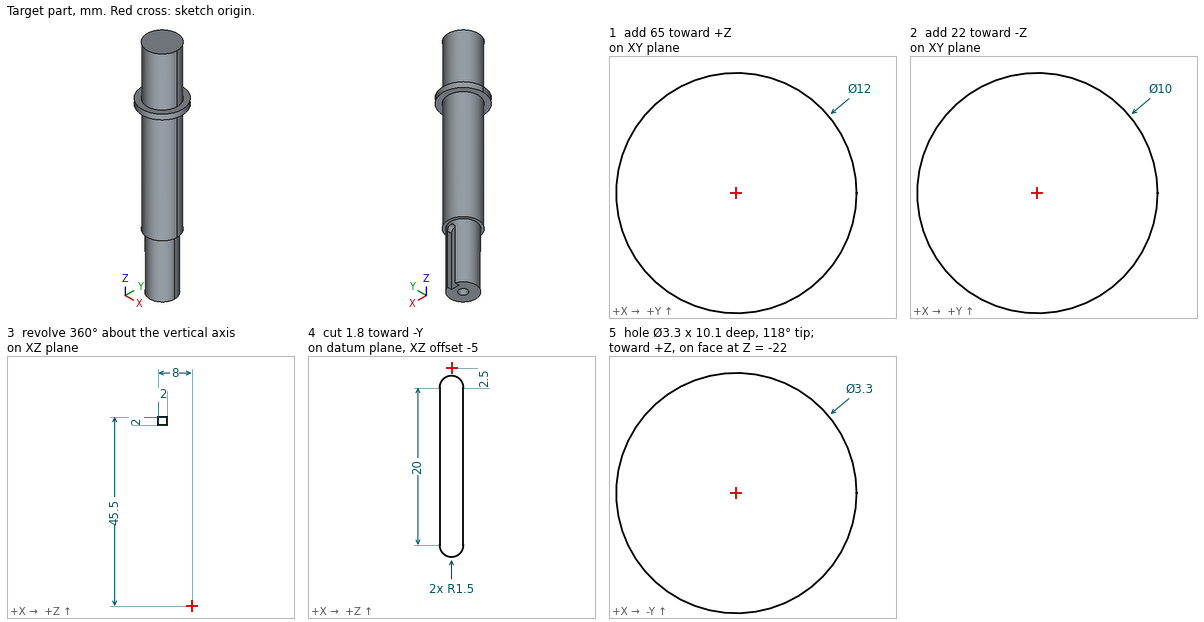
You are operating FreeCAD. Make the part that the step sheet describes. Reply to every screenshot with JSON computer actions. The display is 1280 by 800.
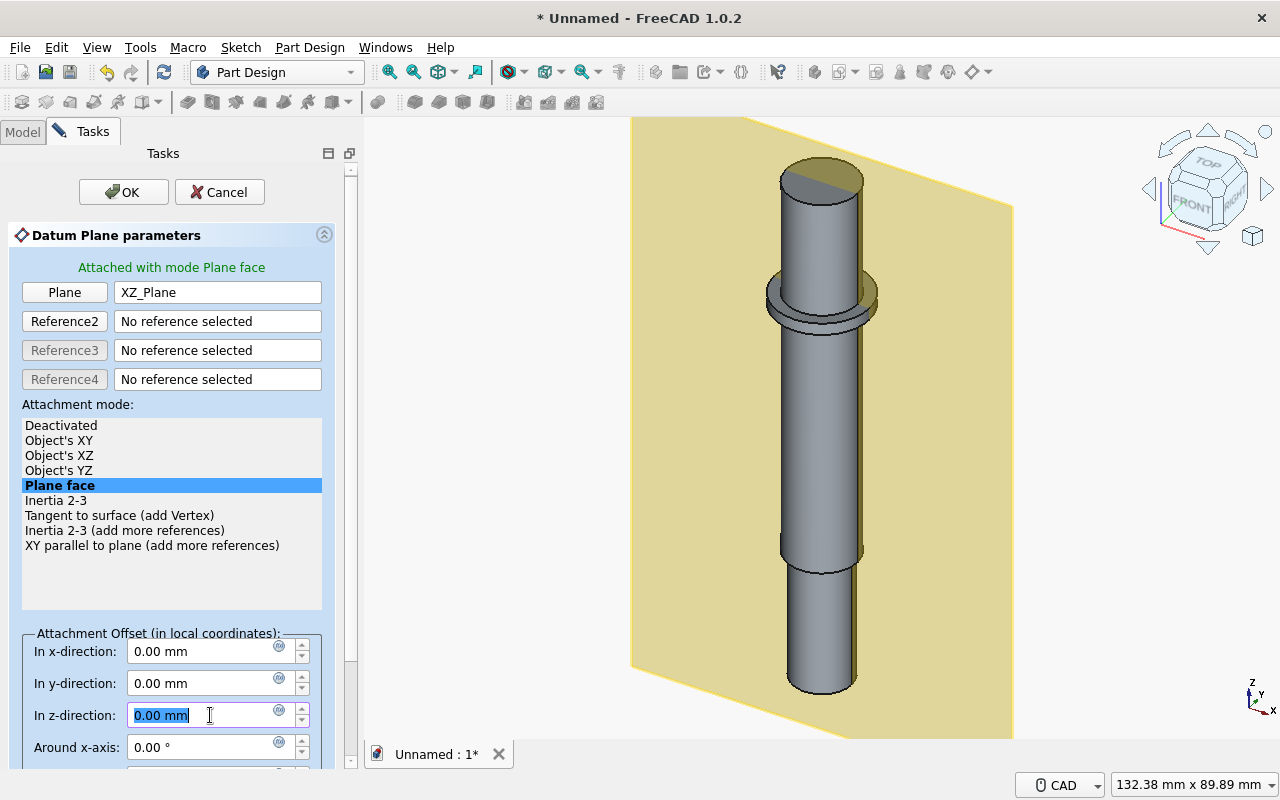
{"action": "type", "text": "-5"}
{"action": "key", "text": "Tab"}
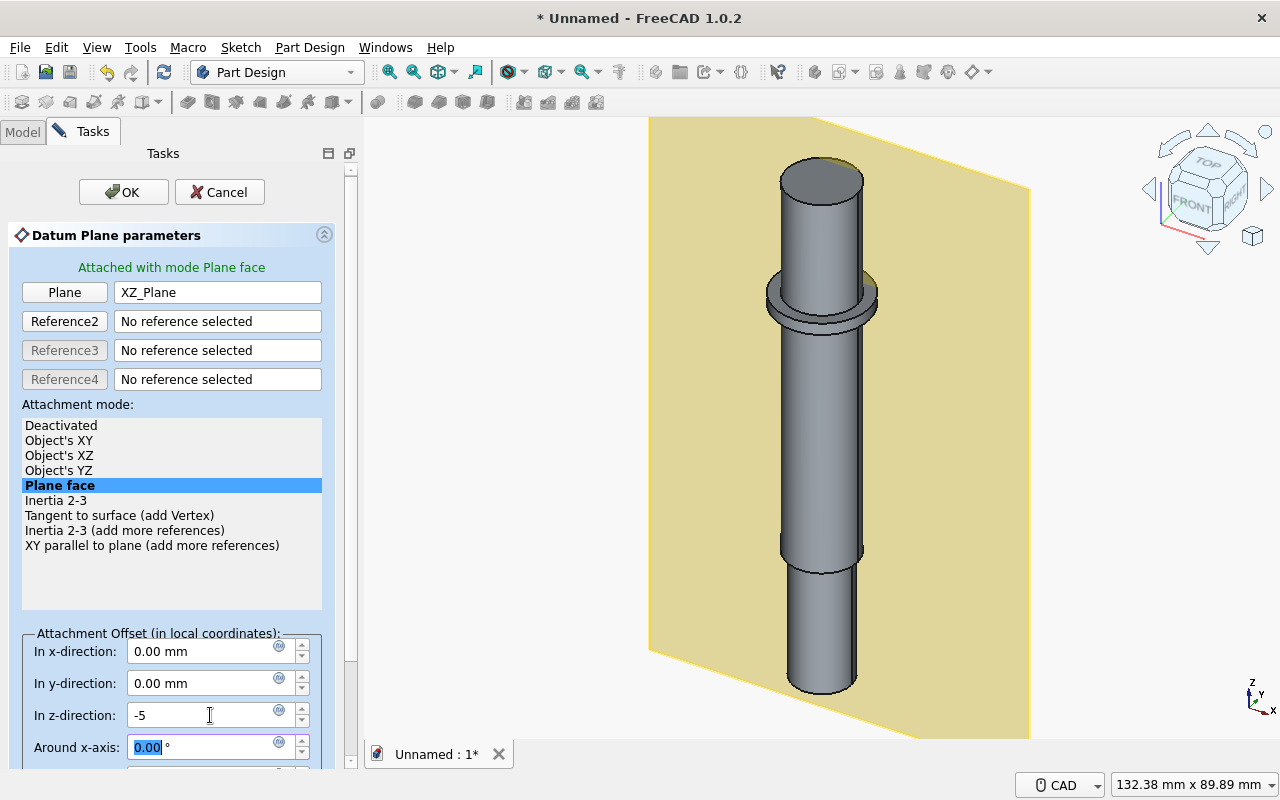
{"action": "left_click", "coordinate": [124, 192]}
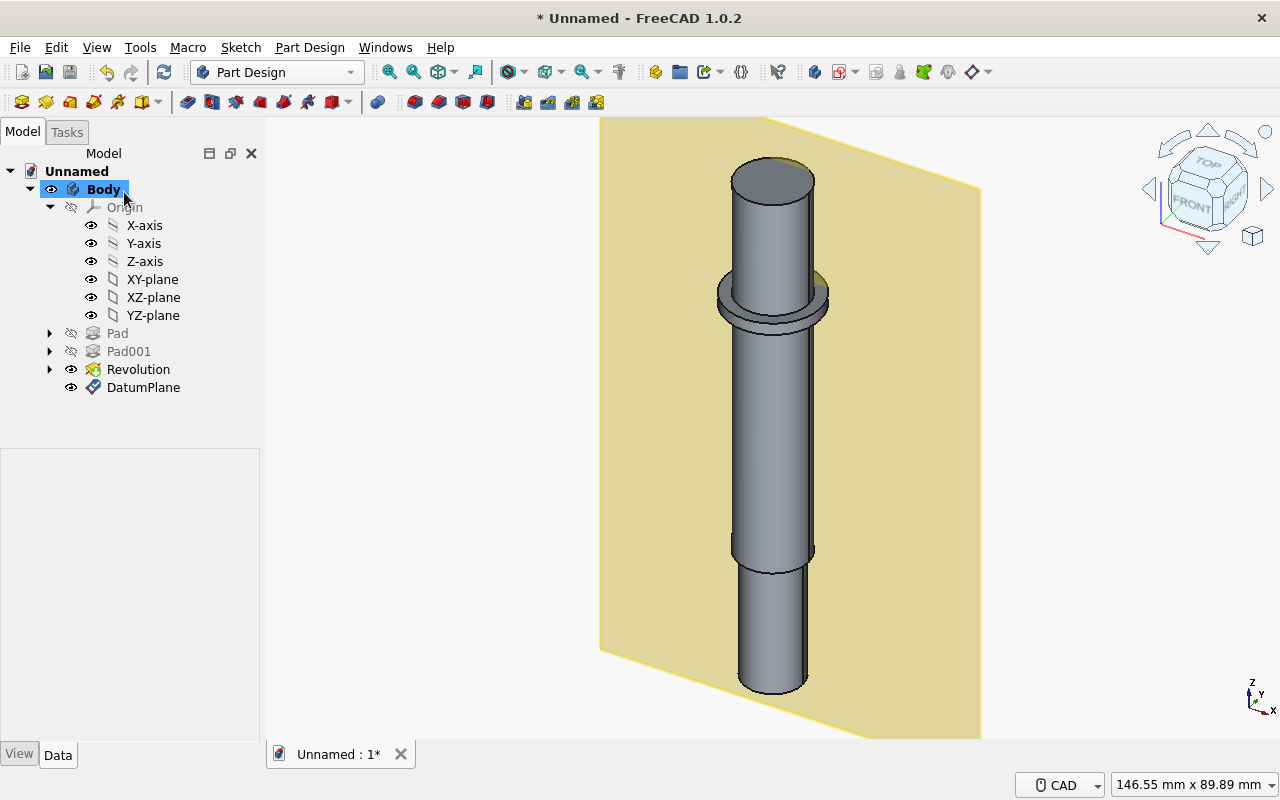
{"action": "left_click", "coordinate": [116, 387]}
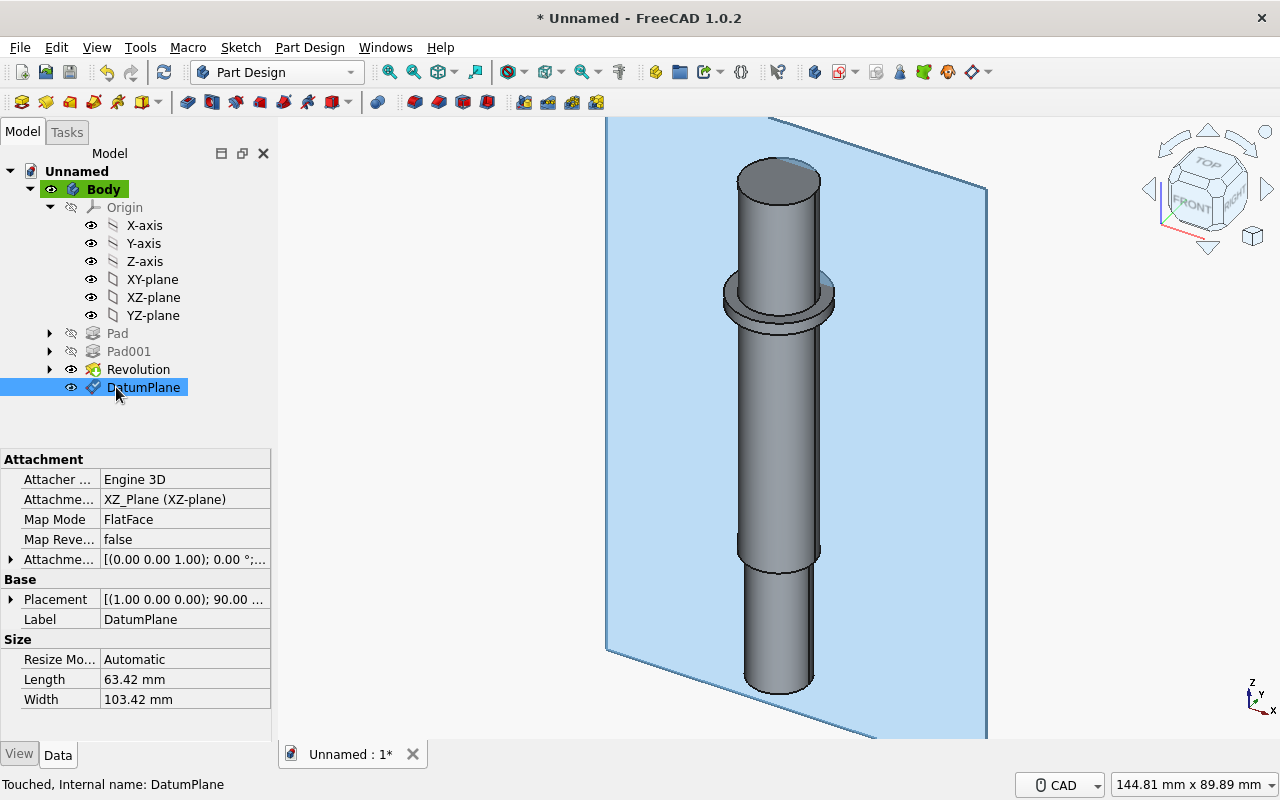
{"action": "left_click", "coordinate": [840, 72]}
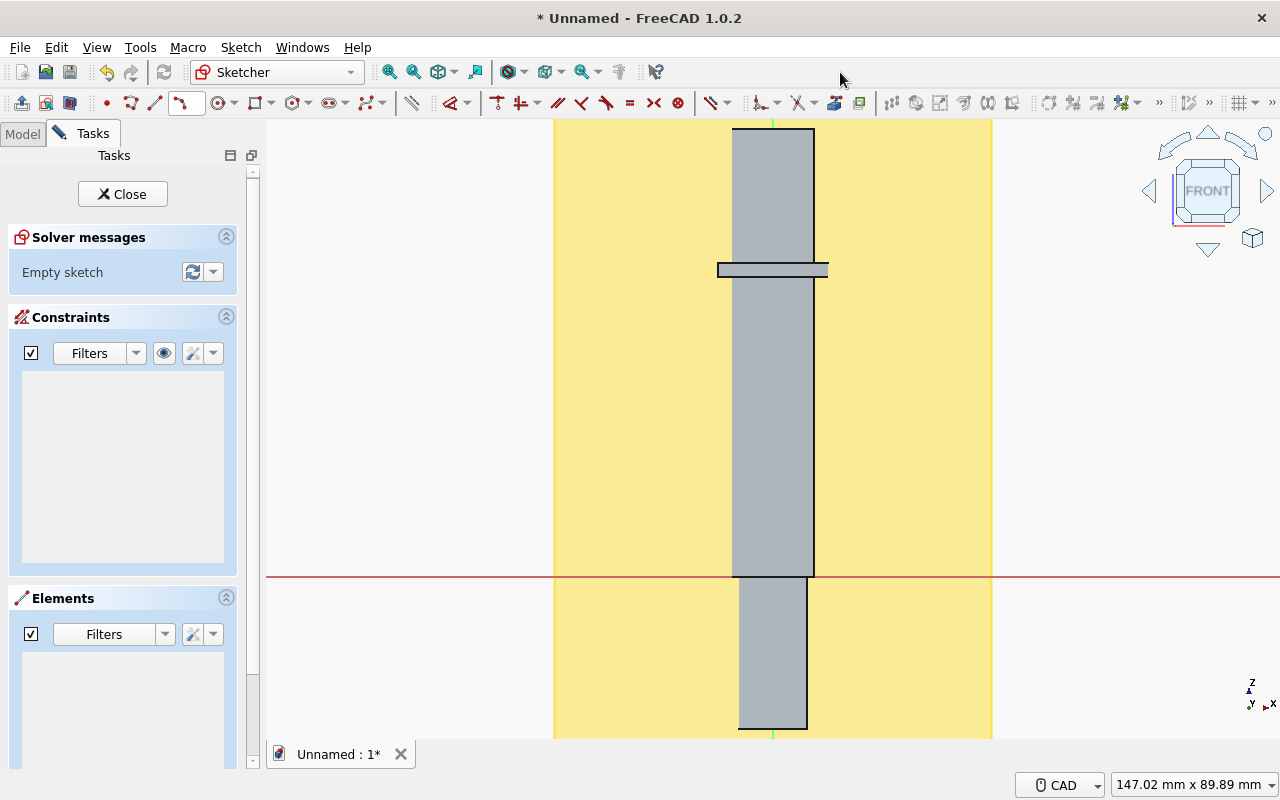
{"action": "left_click", "coordinate": [70, 104]}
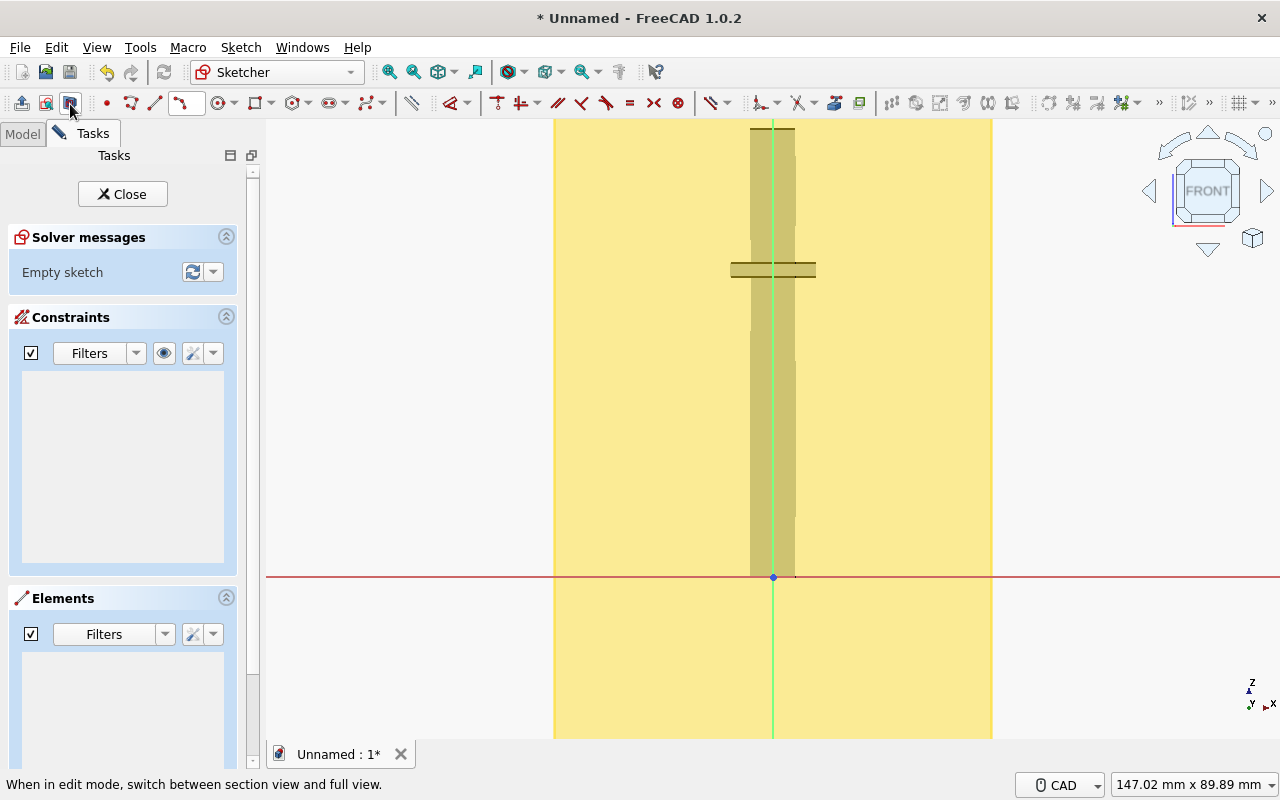
{"action": "scroll", "coordinate": [704, 429], "scroll_direction": "down", "scroll_amount": 5}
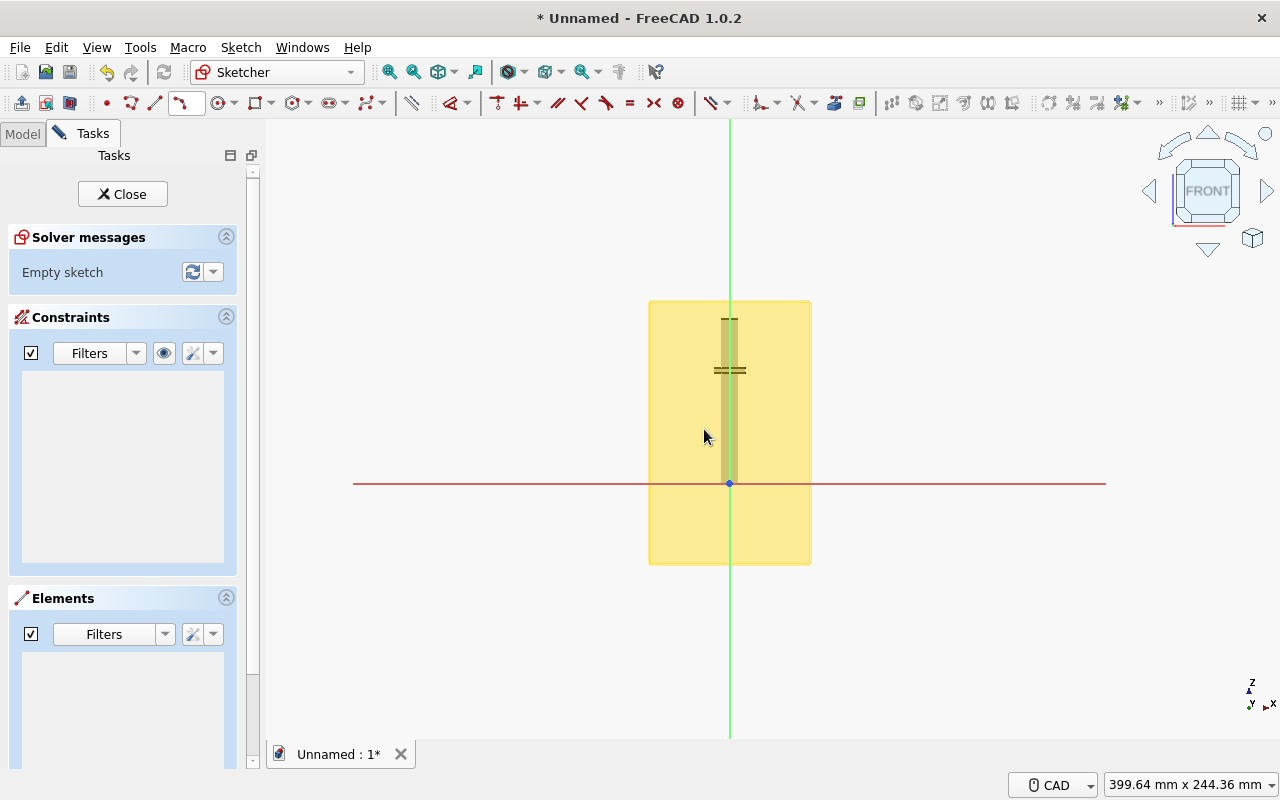
{"action": "scroll", "coordinate": [735, 531], "scroll_direction": "up", "scroll_amount": 9}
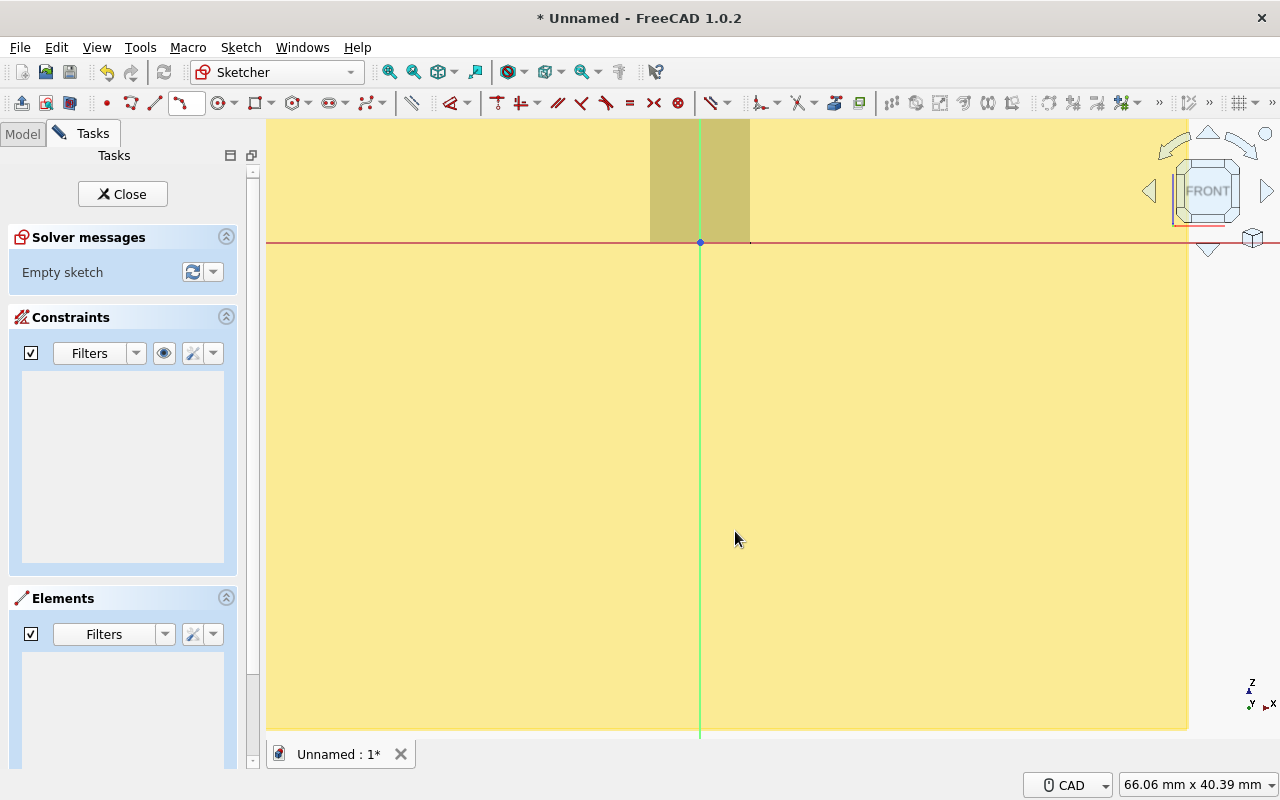
{"action": "left_click", "coordinate": [330, 104]}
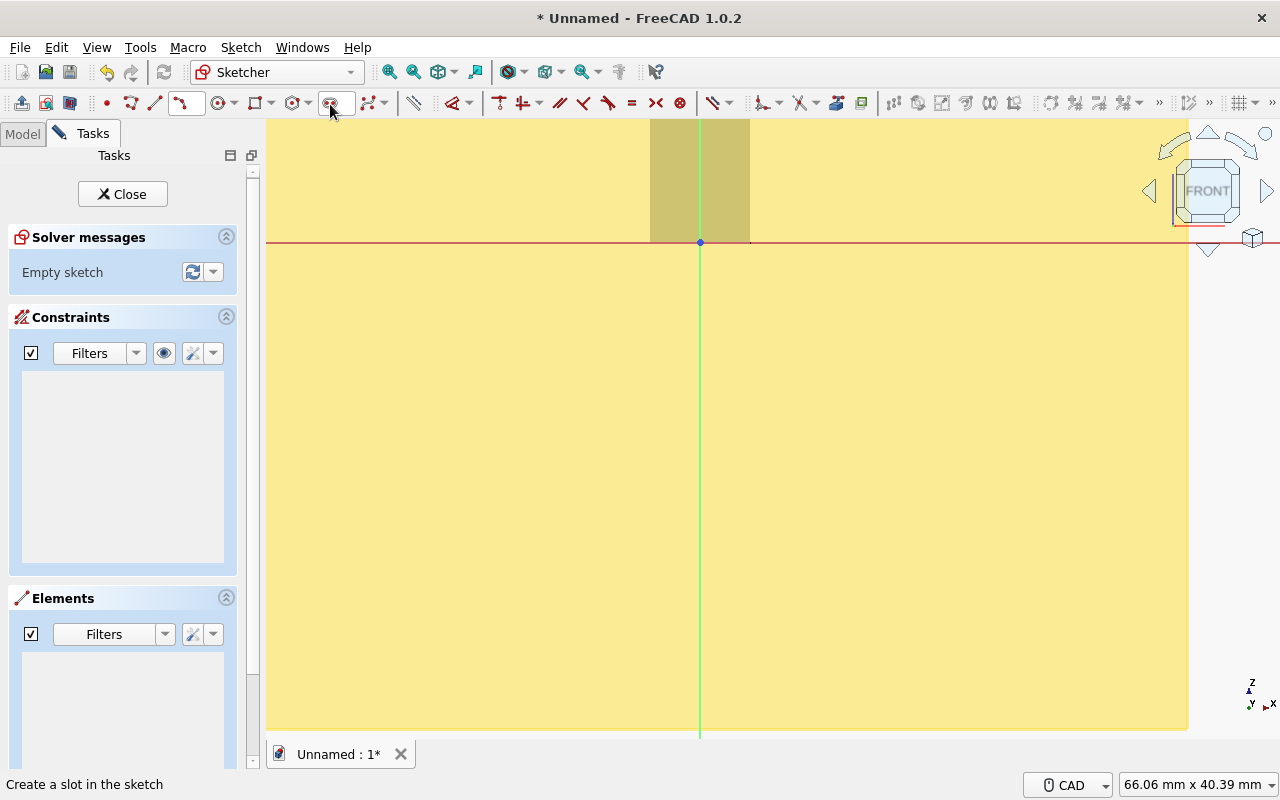
{"action": "left_click", "coordinate": [700, 588]}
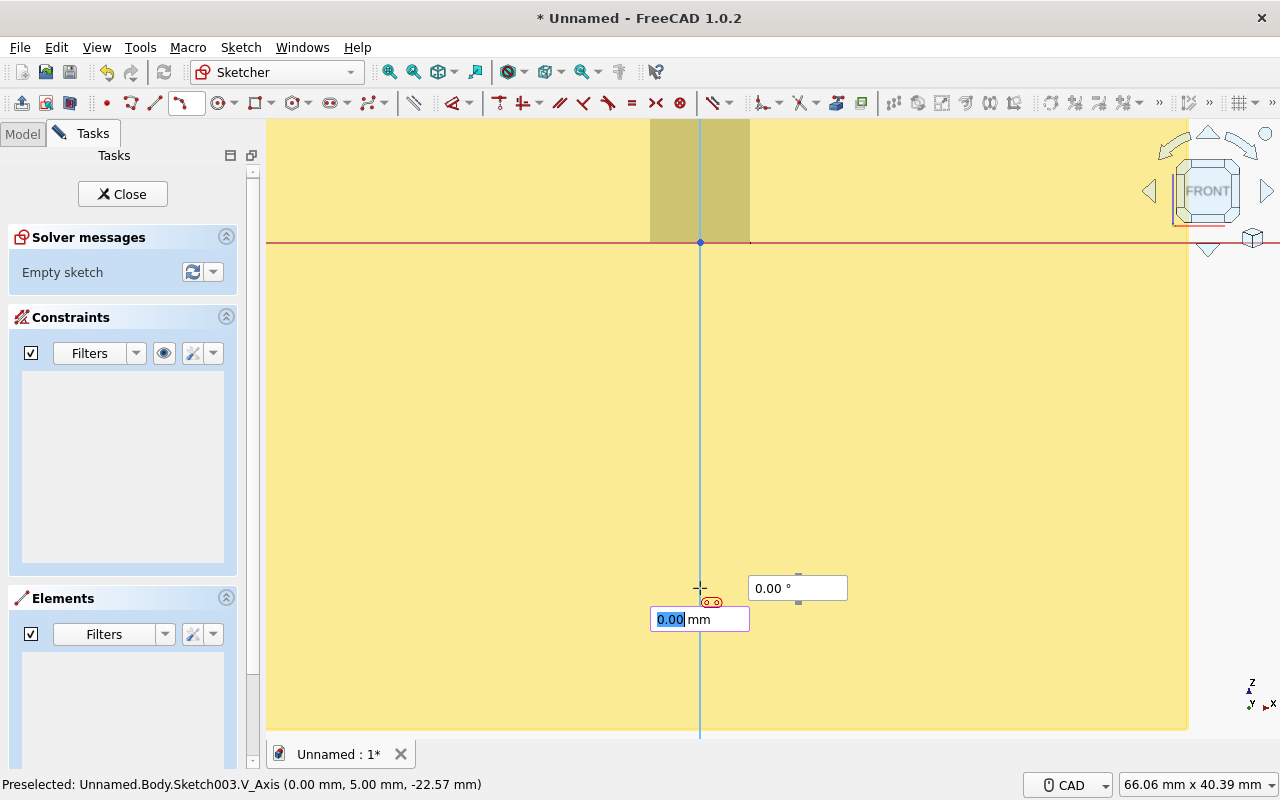
{"action": "left_click", "coordinate": [709, 281]}